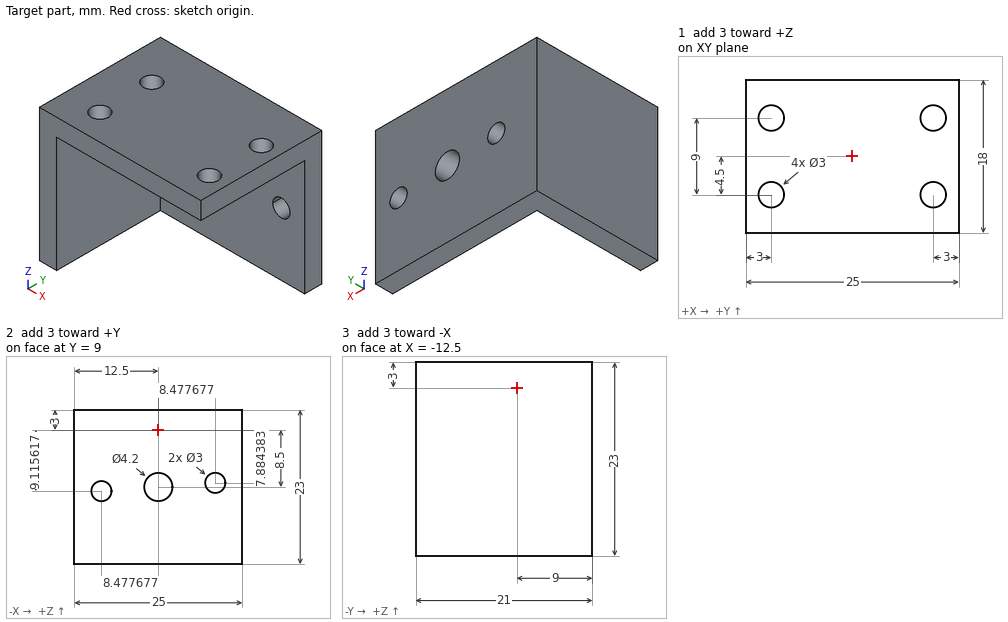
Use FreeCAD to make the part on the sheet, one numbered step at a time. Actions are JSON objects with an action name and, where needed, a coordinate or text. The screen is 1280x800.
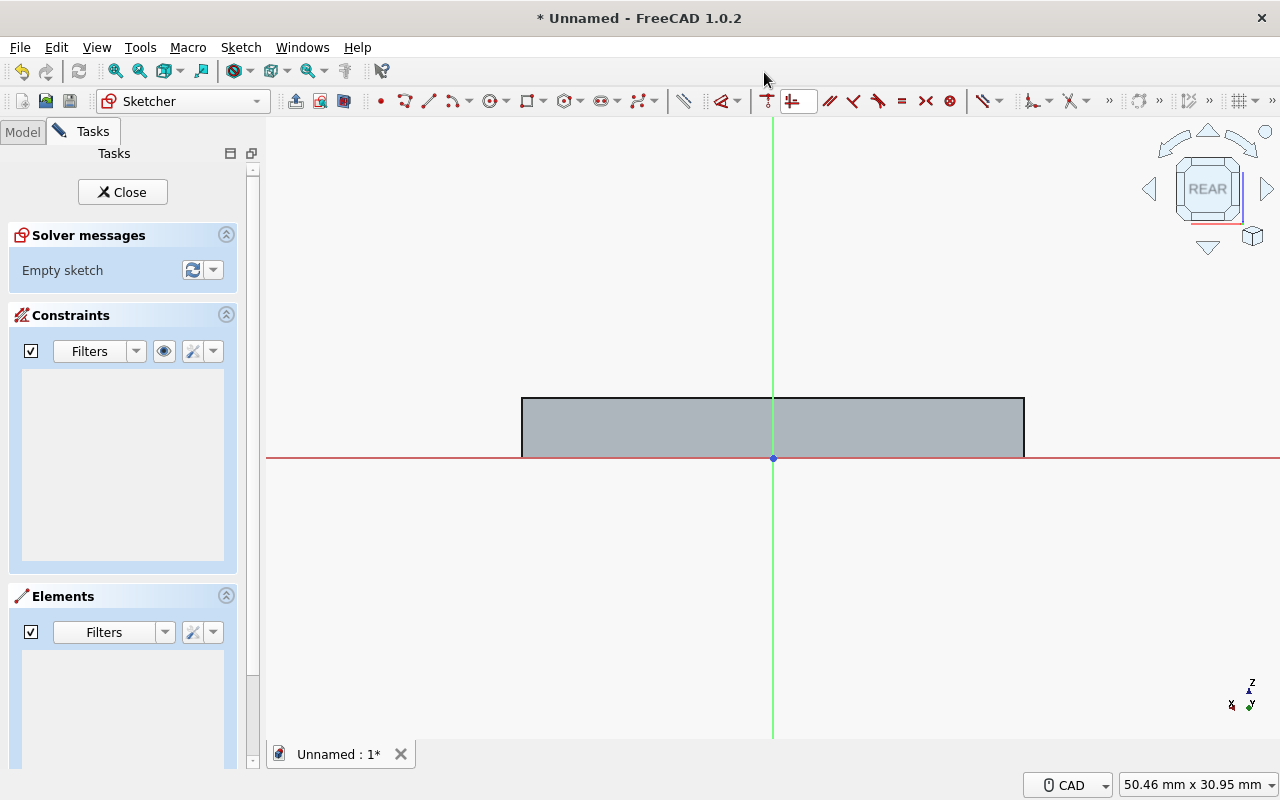
{"action": "scroll", "coordinate": [565, 145], "scroll_direction": "down", "scroll_amount": 2}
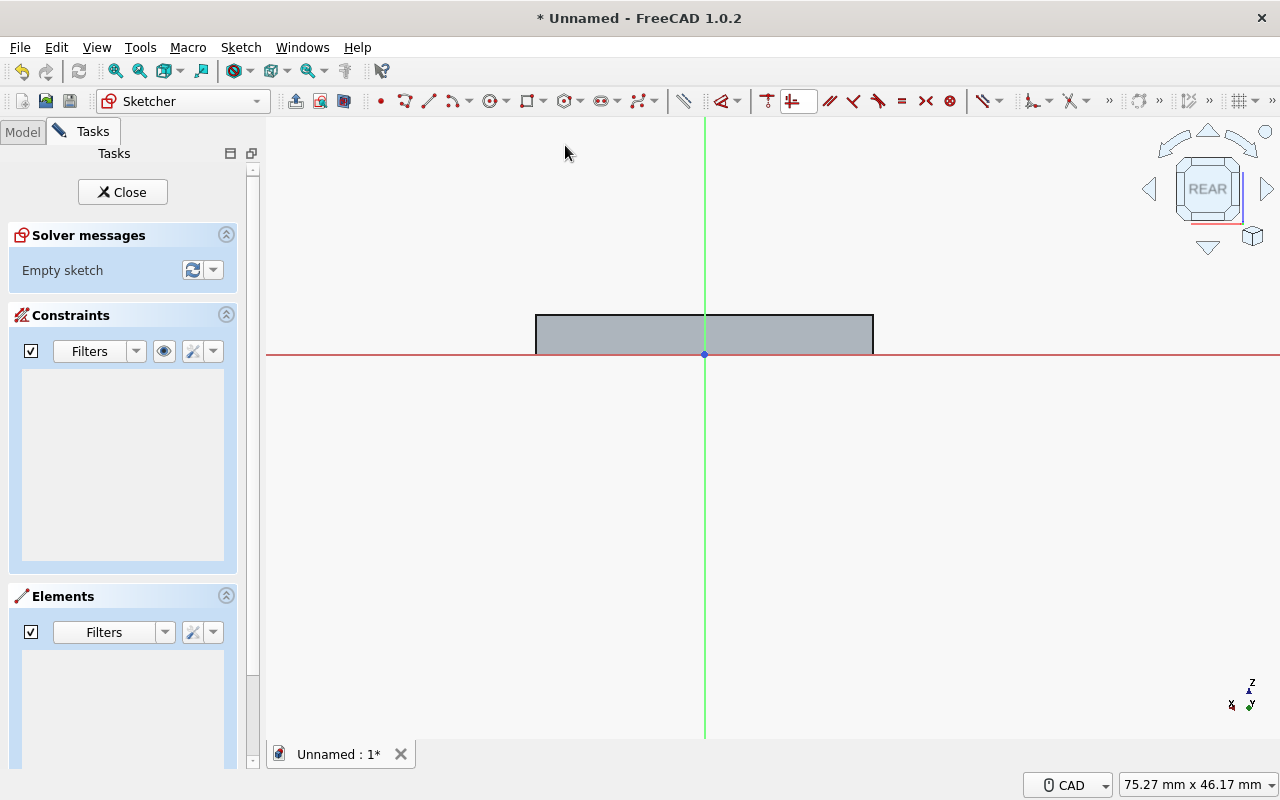
{"action": "key", "text": "g r"}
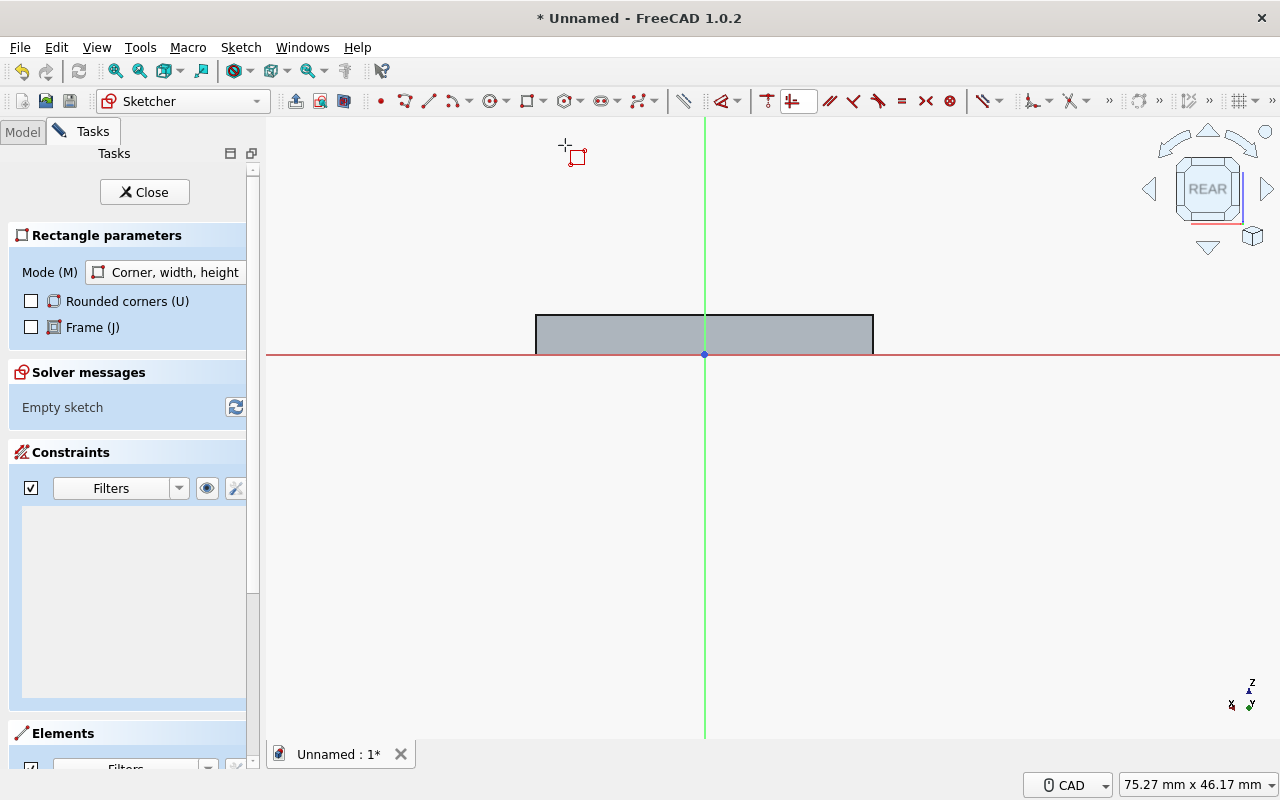
{"action": "left_click", "coordinate": [536, 315]}
{"action": "mouse_move", "coordinate": [873, 624]}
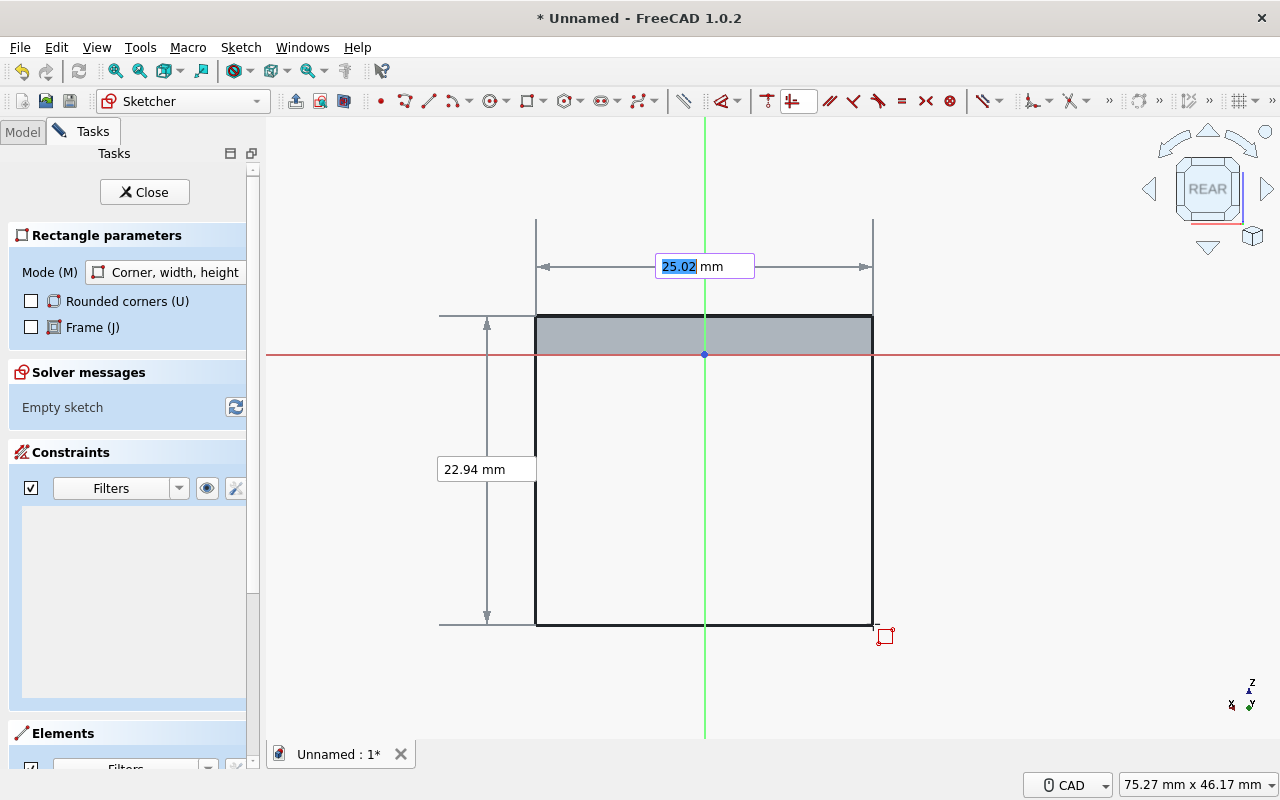
{"action": "type", "text": "25"}
{"action": "key", "text": "Tab"}
{"action": "type", "text": "23"}
{"action": "key", "text": "Return"}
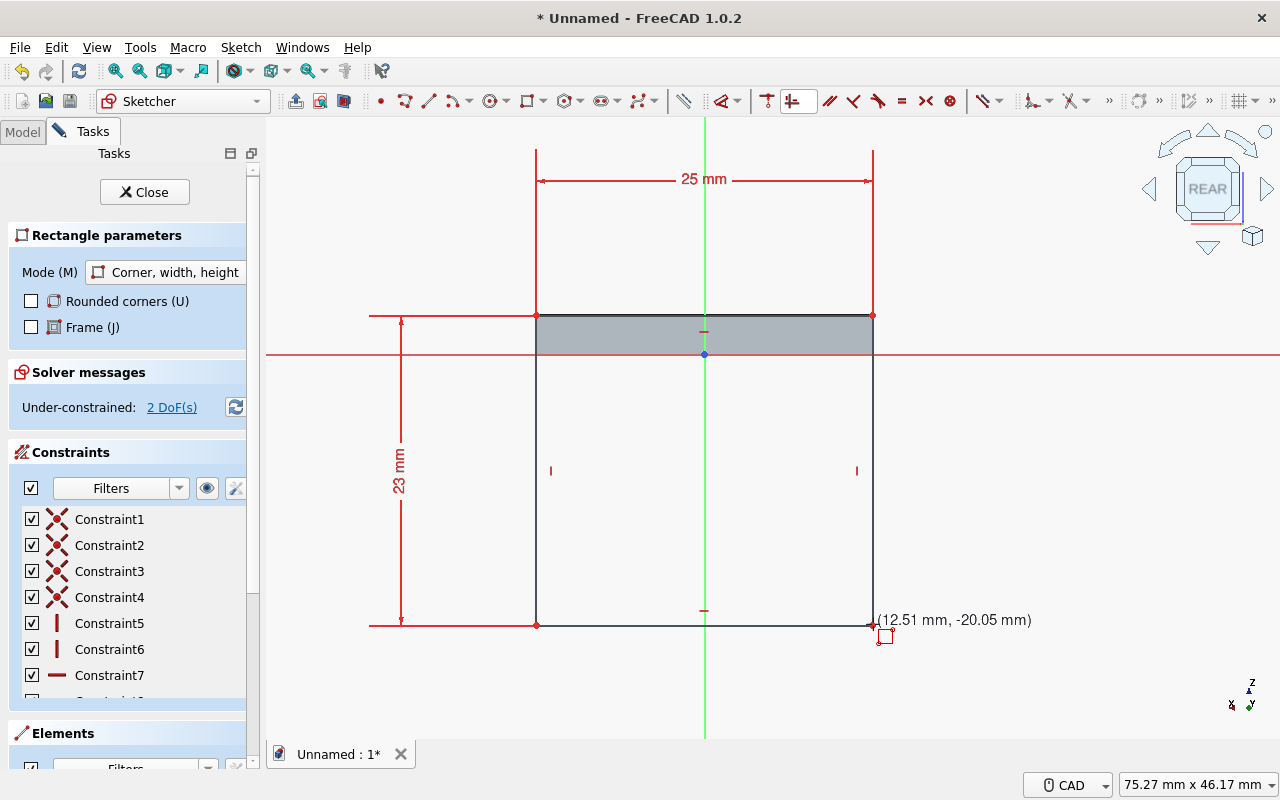
{"action": "key", "text": "g c"}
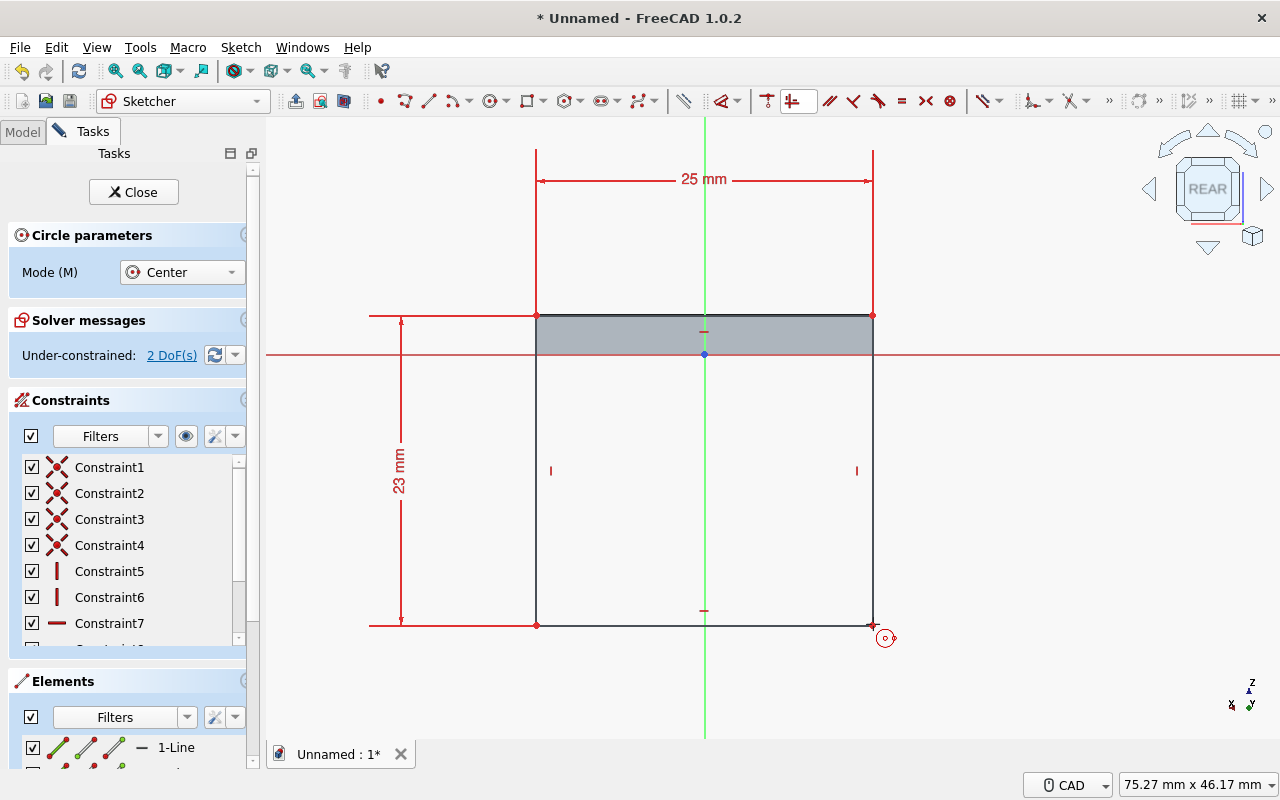
{"action": "left_click", "coordinate": [819, 461]}
{"action": "mouse_move", "coordinate": [833, 447]}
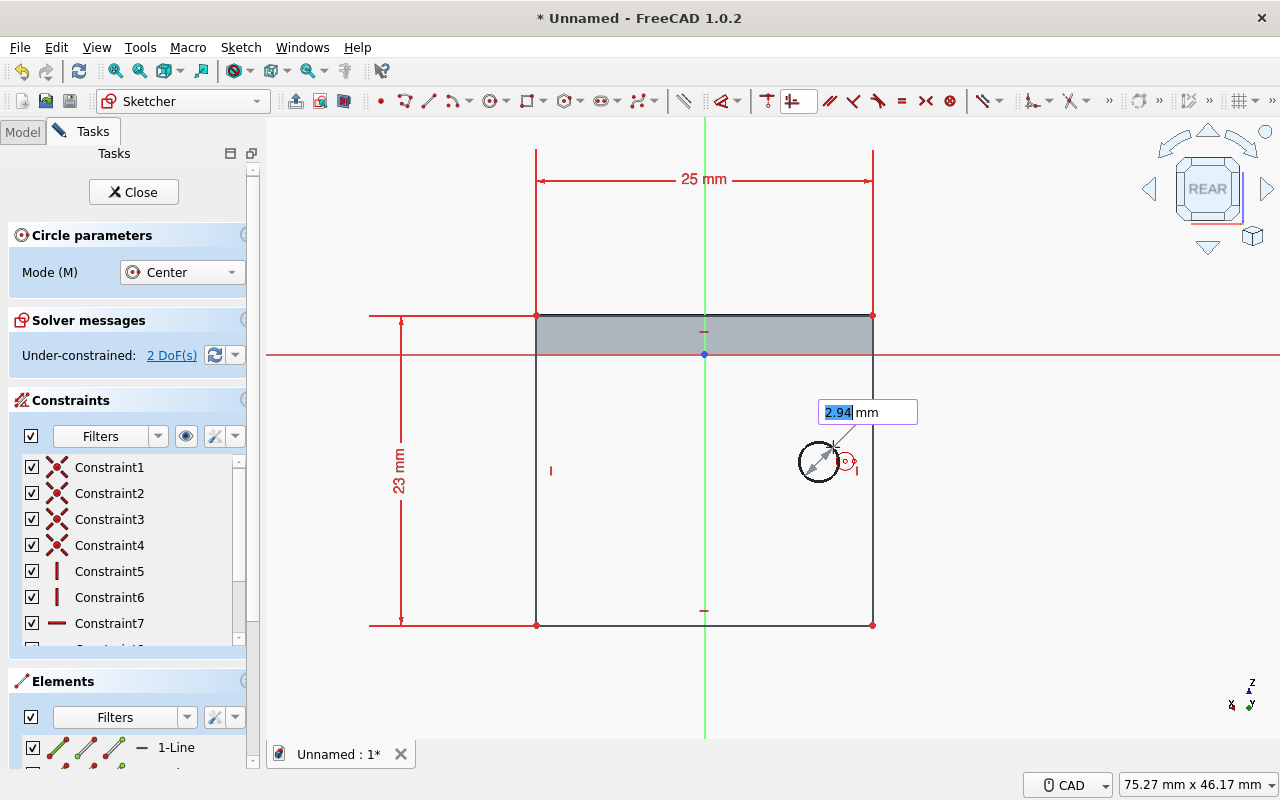
{"action": "type", "text": "3"}
{"action": "key", "text": "Return"}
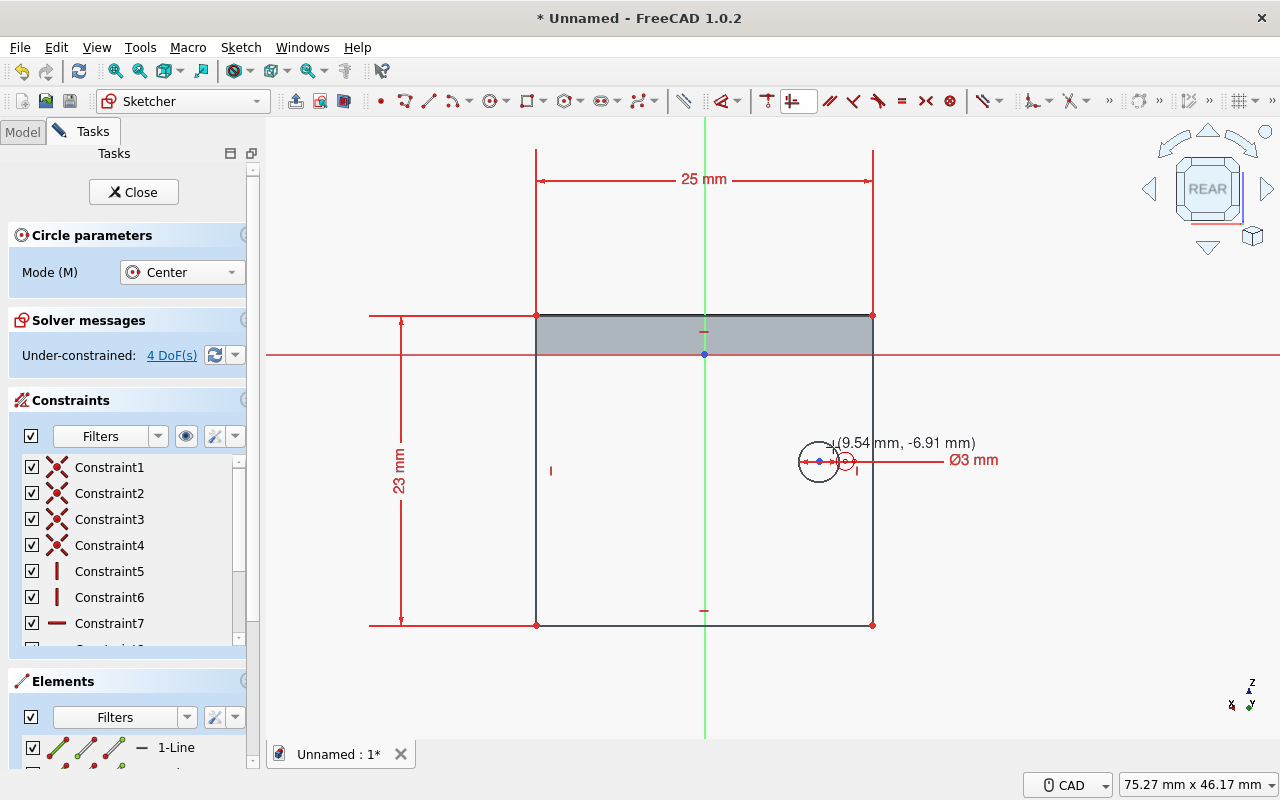
{"action": "left_click", "coordinate": [705, 469]}
{"action": "mouse_move", "coordinate": [725, 449]}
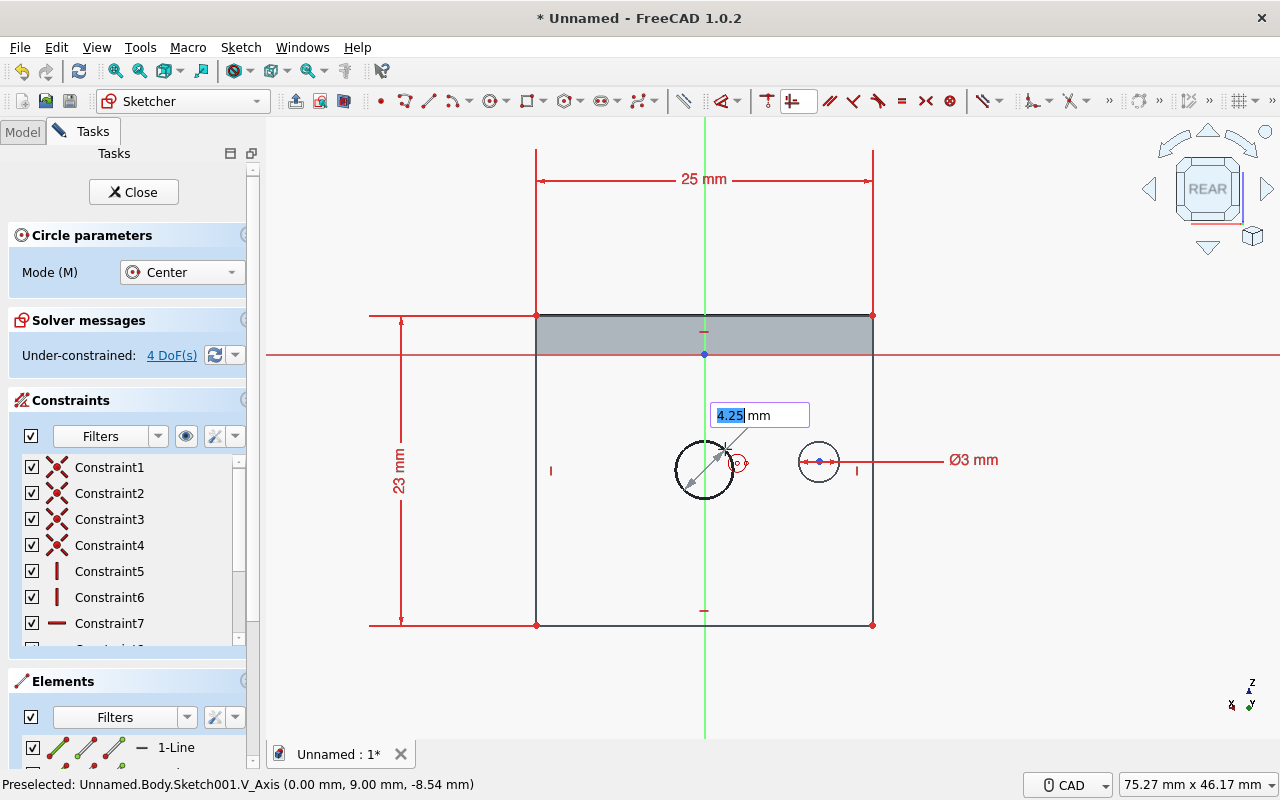
{"action": "type", "text": "4.2"}
{"action": "key", "text": "Return"}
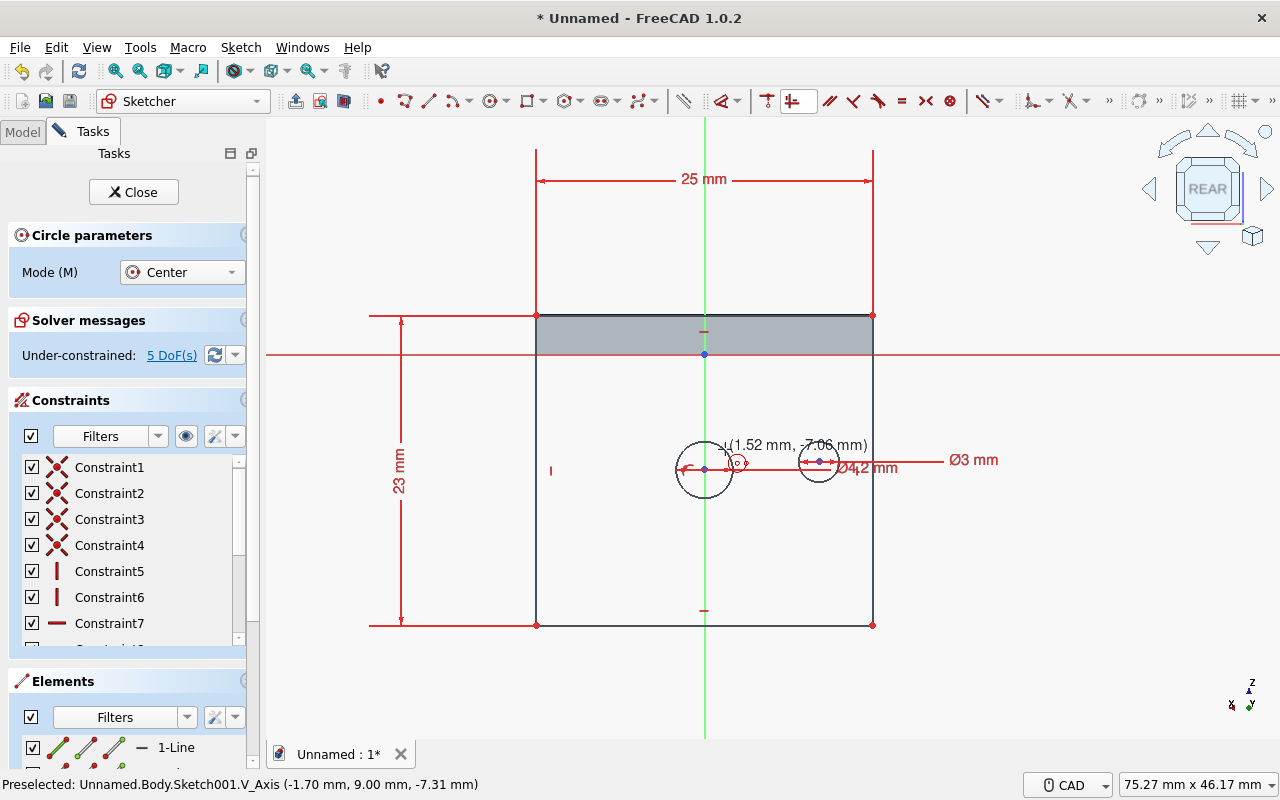
{"action": "left_click", "coordinate": [590, 478]}
{"action": "mouse_move", "coordinate": [605, 463]}